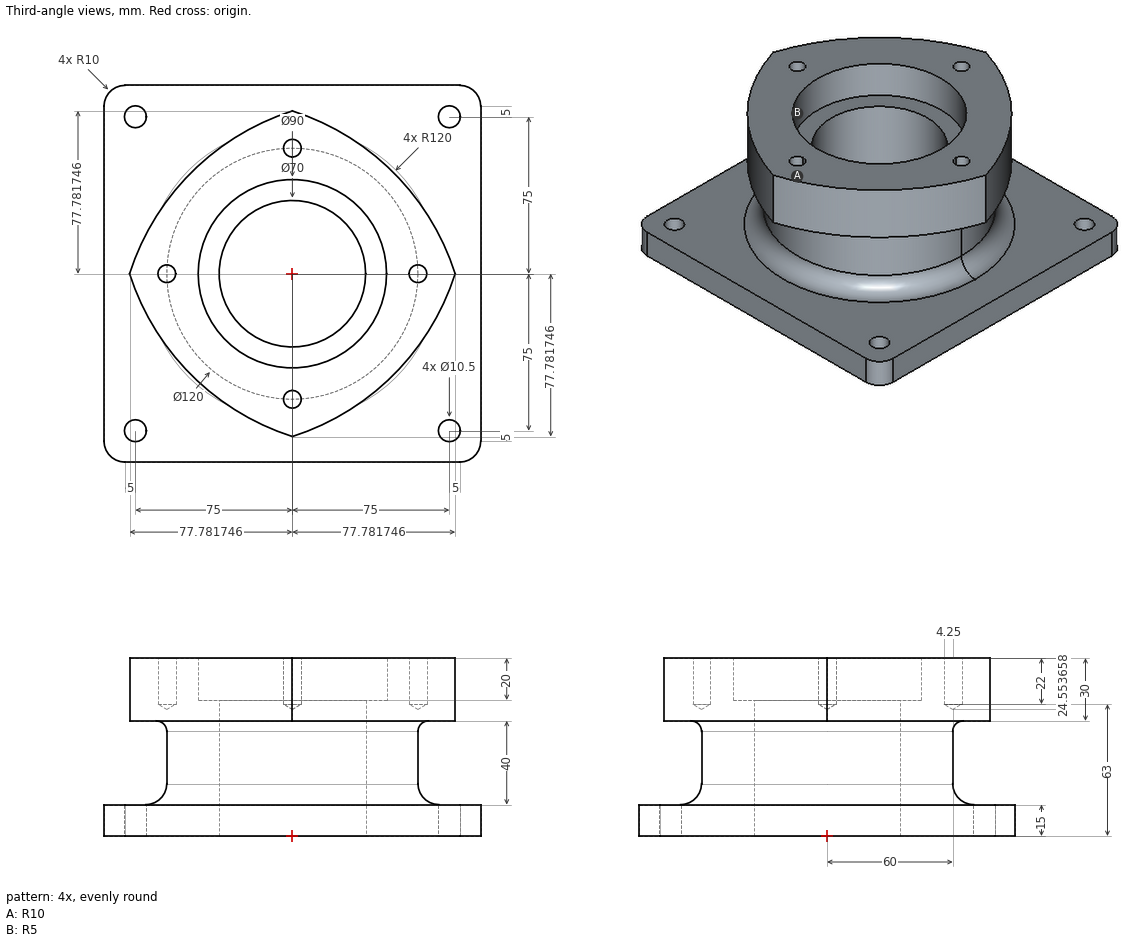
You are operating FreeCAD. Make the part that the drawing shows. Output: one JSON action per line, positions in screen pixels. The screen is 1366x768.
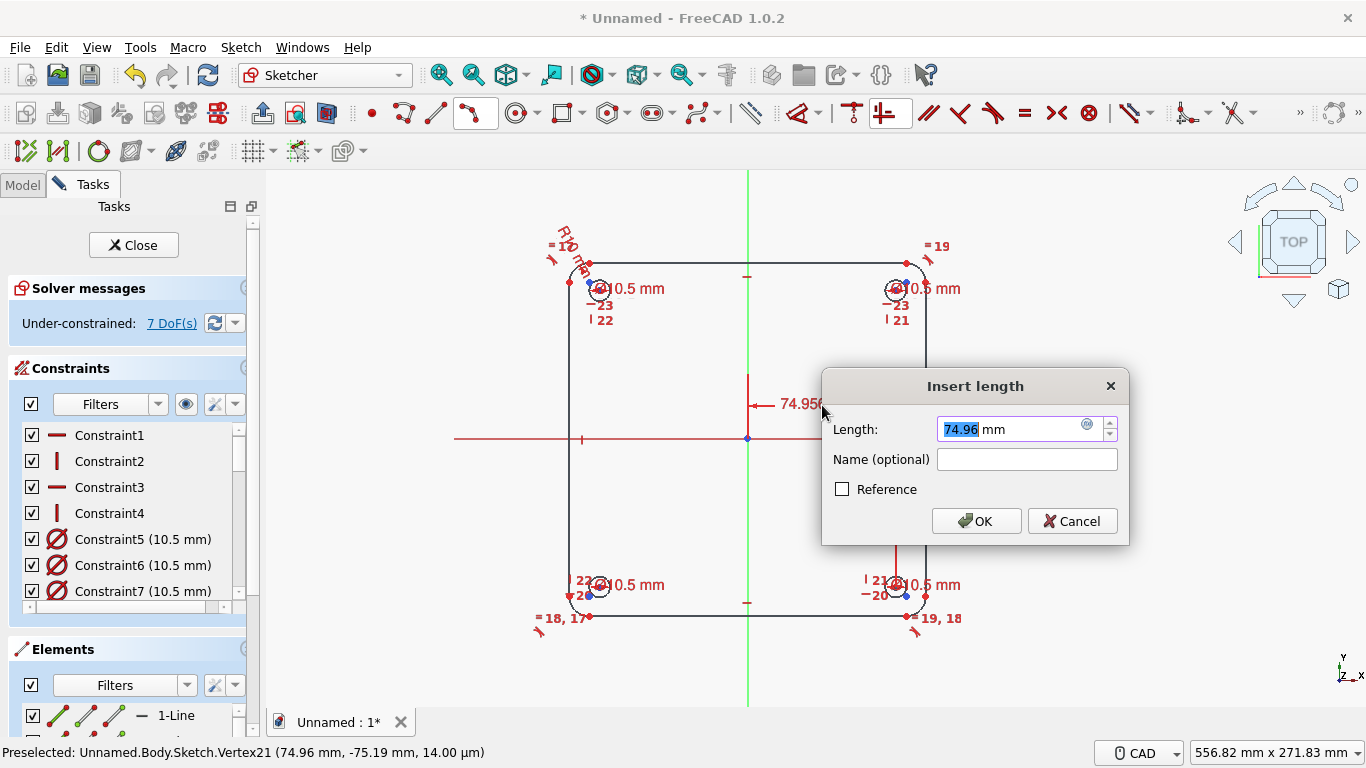
{"action": "type", "text": "75"}
{"action": "key", "text": "Return"}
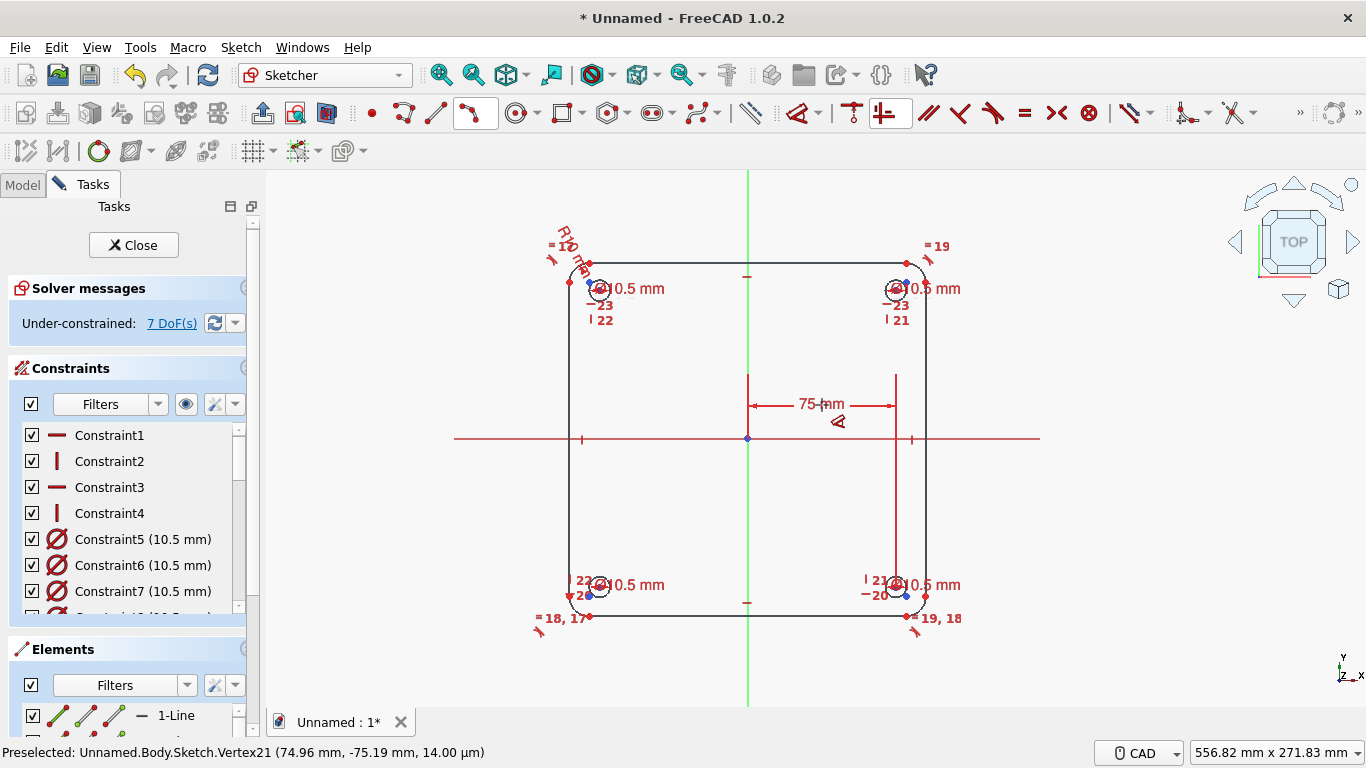
{"action": "left_click", "coordinate": [896, 587]}
{"action": "left_click", "coordinate": [714, 513]}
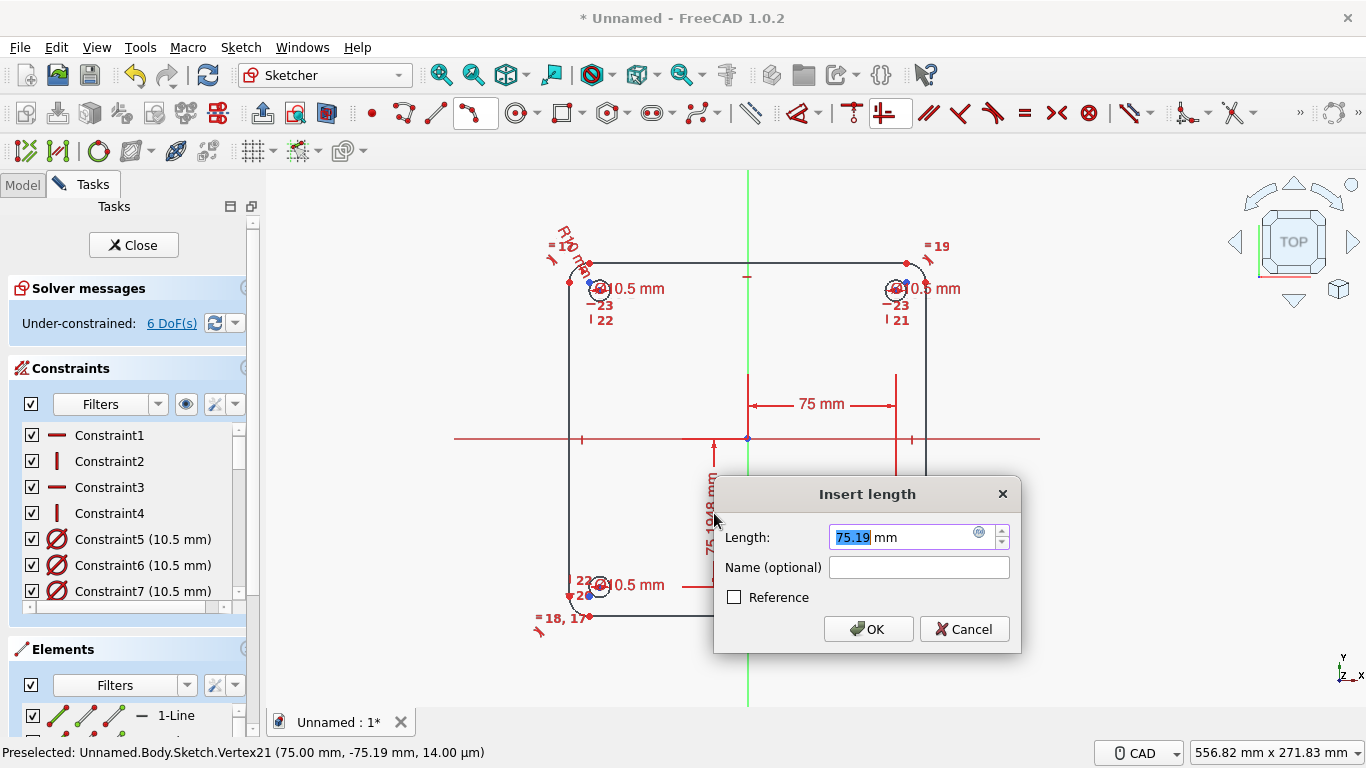
{"action": "type", "text": "75"}
{"action": "key", "text": "Return"}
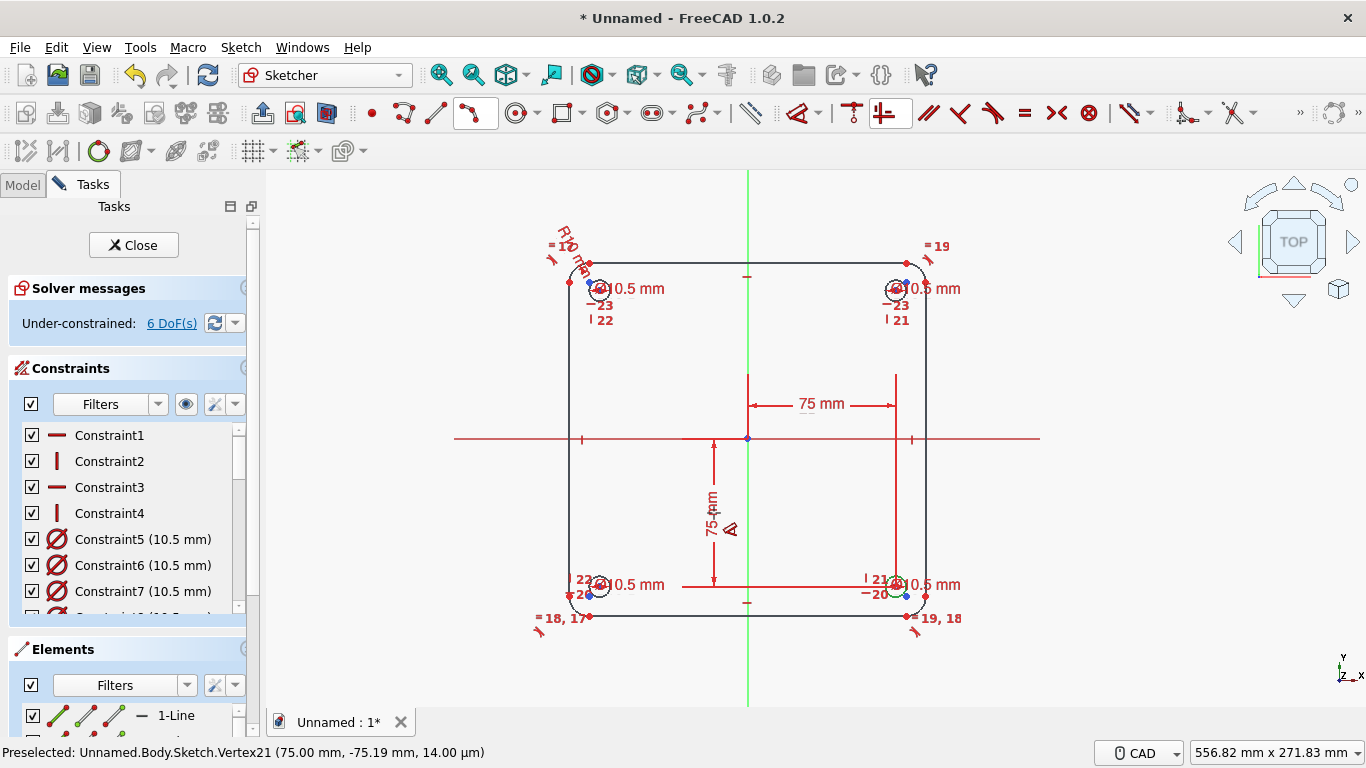
{"action": "left_click", "coordinate": [600, 587]}
{"action": "left_click", "coordinate": [674, 405]}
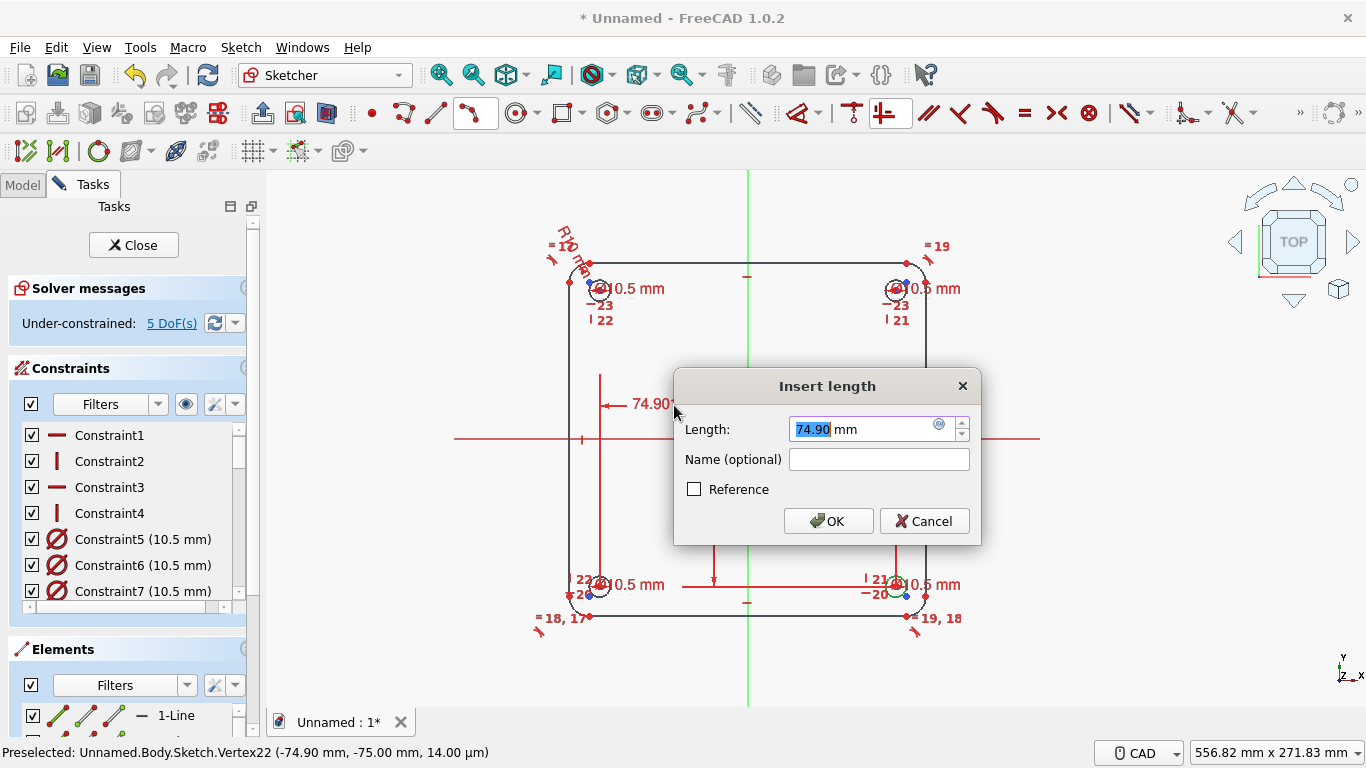
{"action": "type", "text": "75"}
{"action": "key", "text": "Return"}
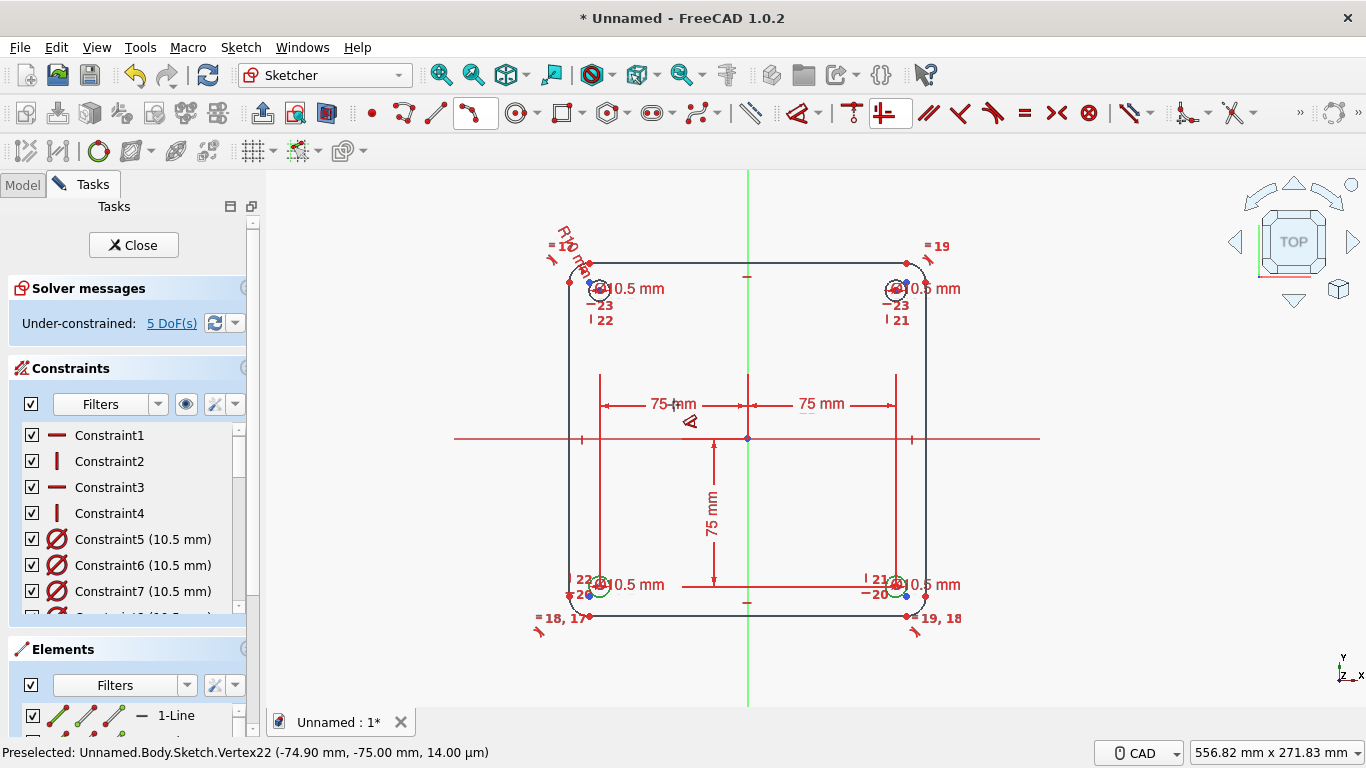
{"action": "left_click", "coordinate": [896, 291]}
{"action": "left_click", "coordinate": [714, 365]}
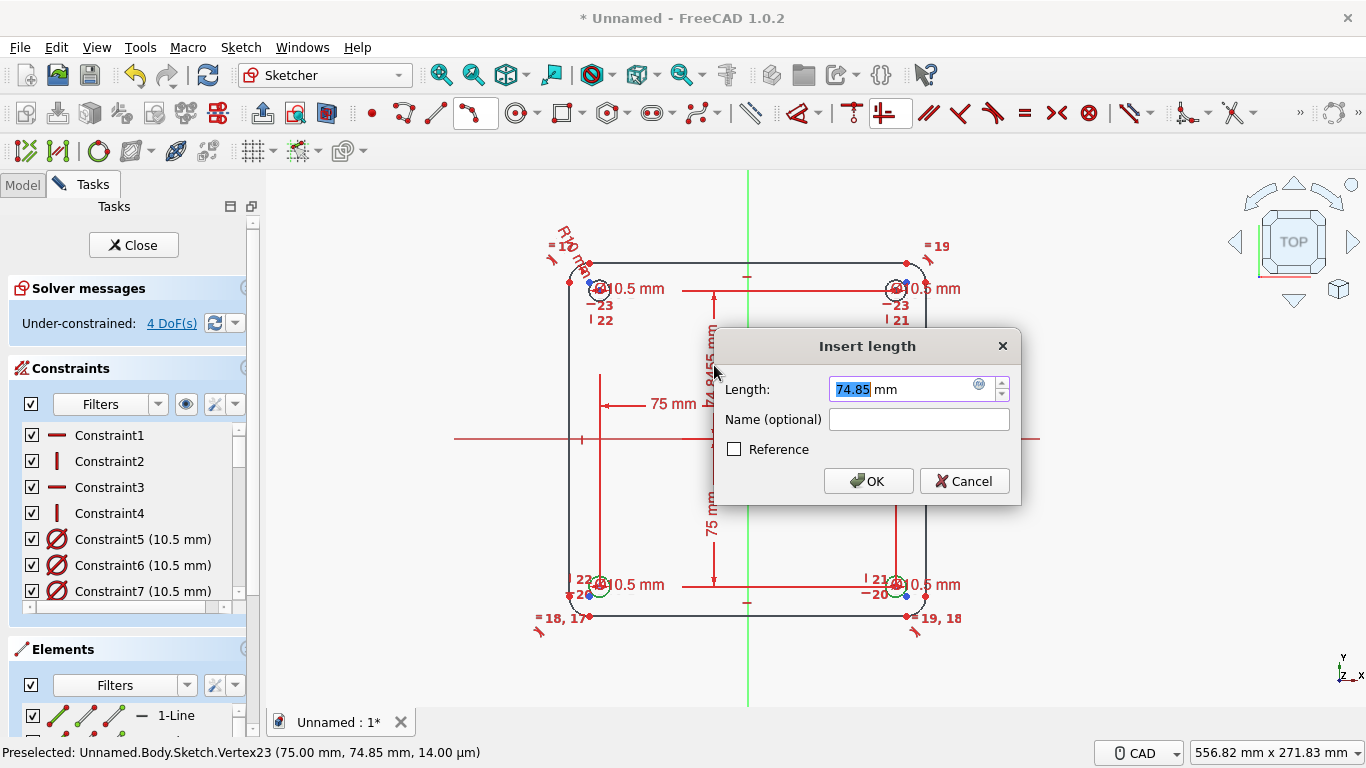
{"action": "type", "text": "75"}
{"action": "key", "text": "Return"}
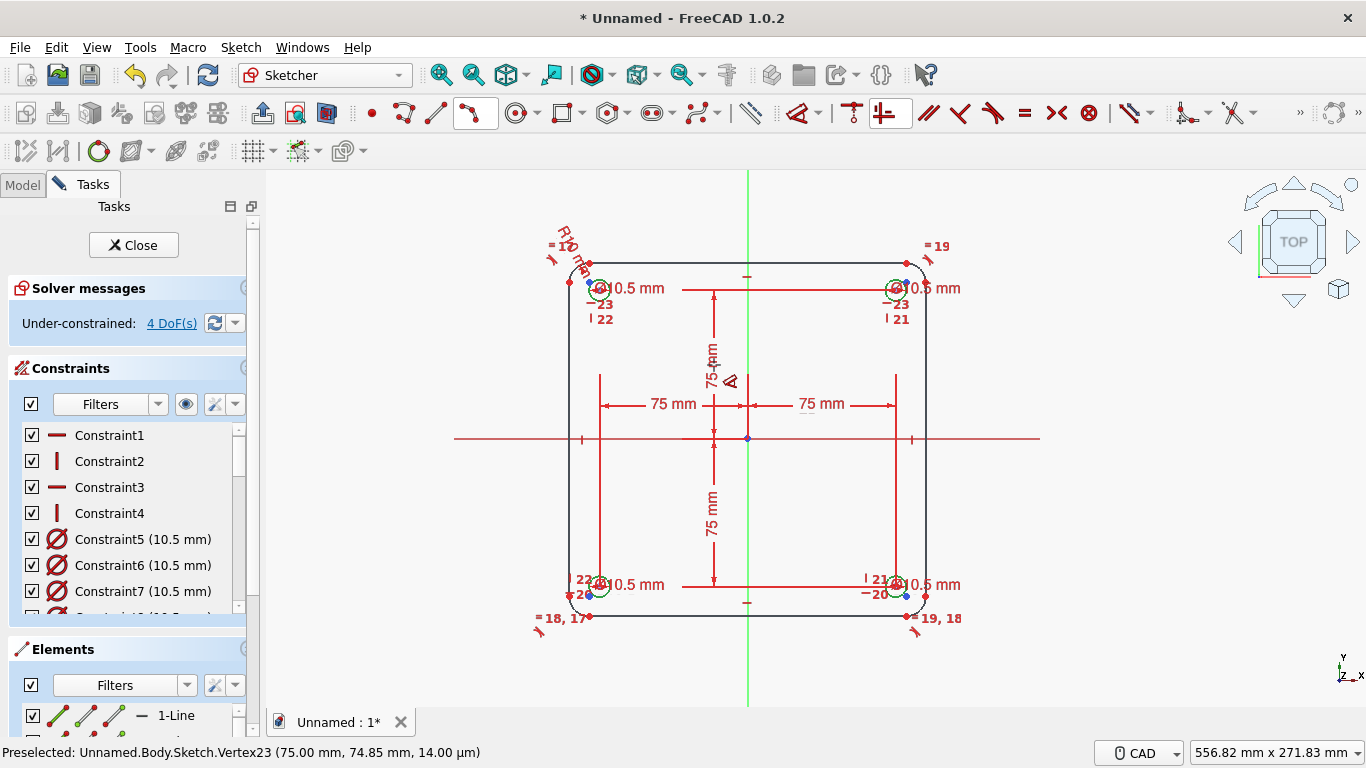
{"action": "scroll", "coordinate": [906, 616], "scroll_direction": "up", "scroll_amount": 7}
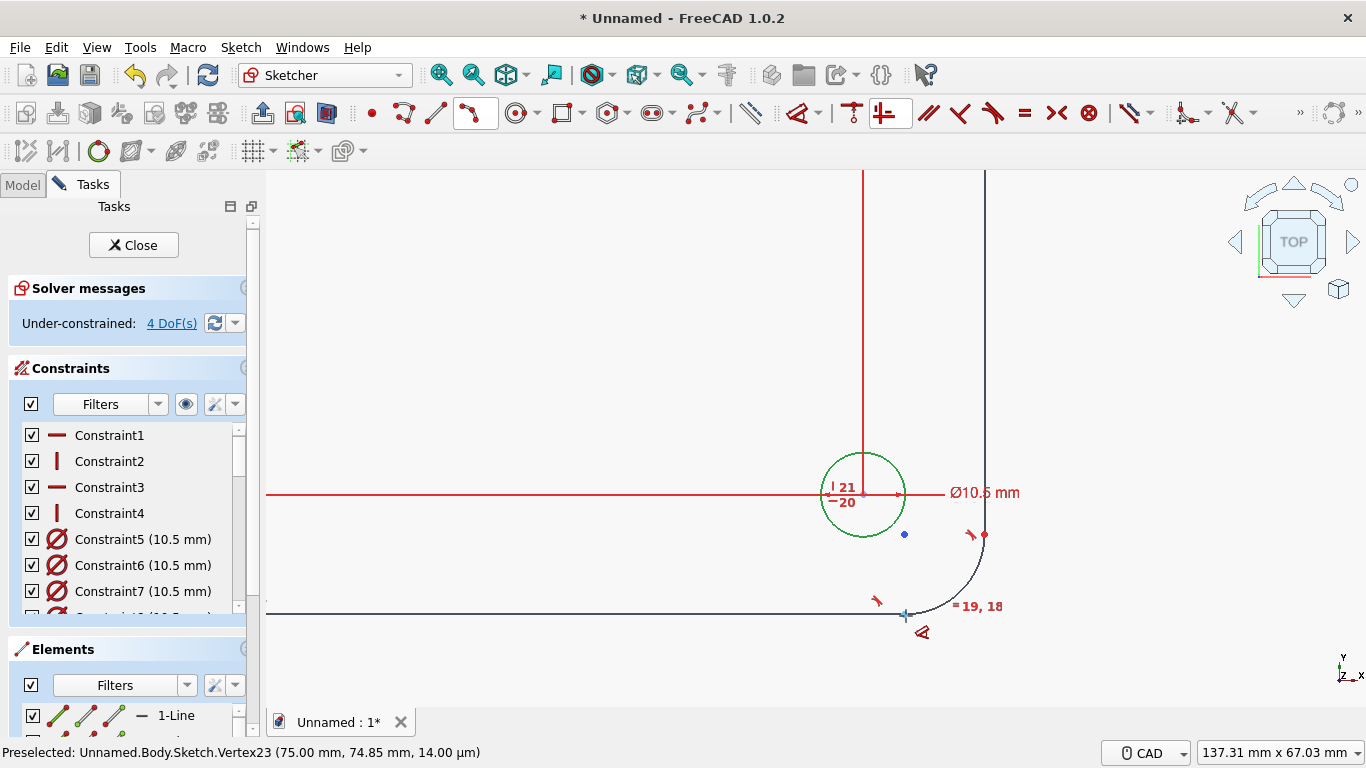
{"action": "left_click", "coordinate": [904, 614]}